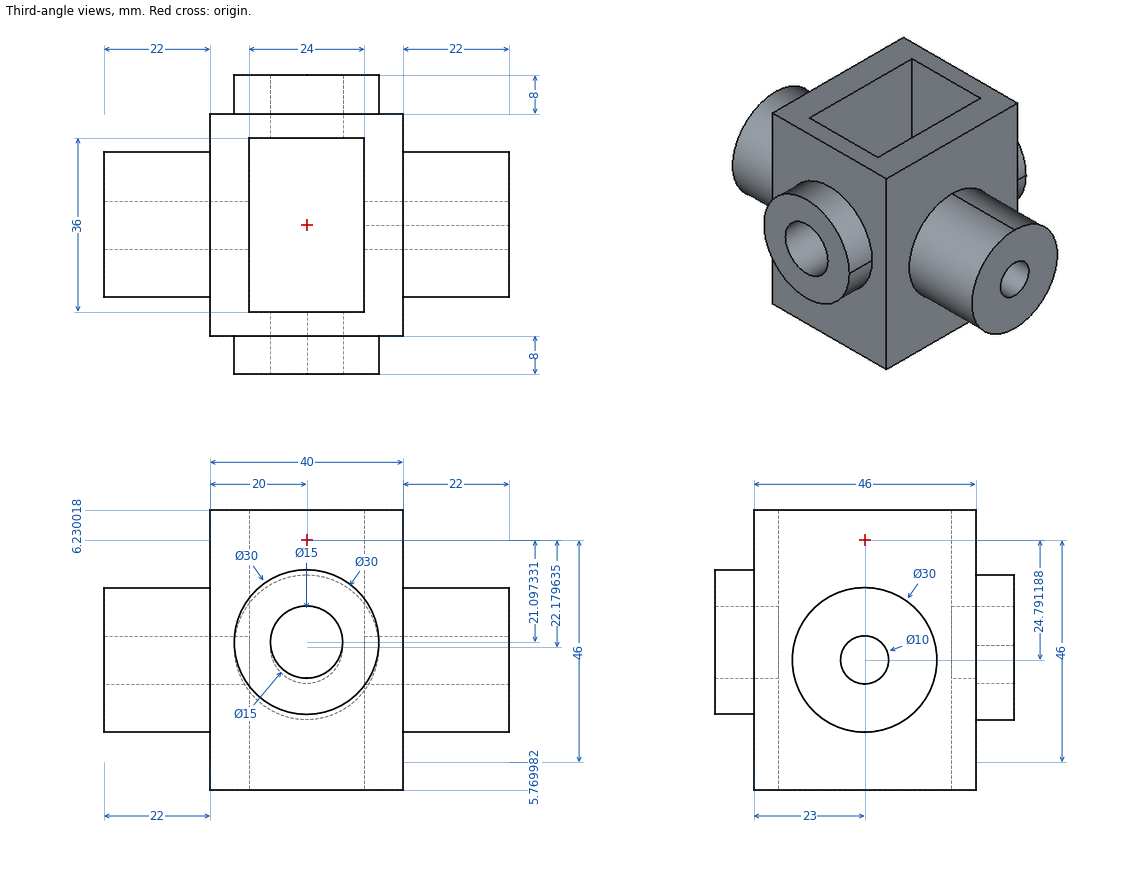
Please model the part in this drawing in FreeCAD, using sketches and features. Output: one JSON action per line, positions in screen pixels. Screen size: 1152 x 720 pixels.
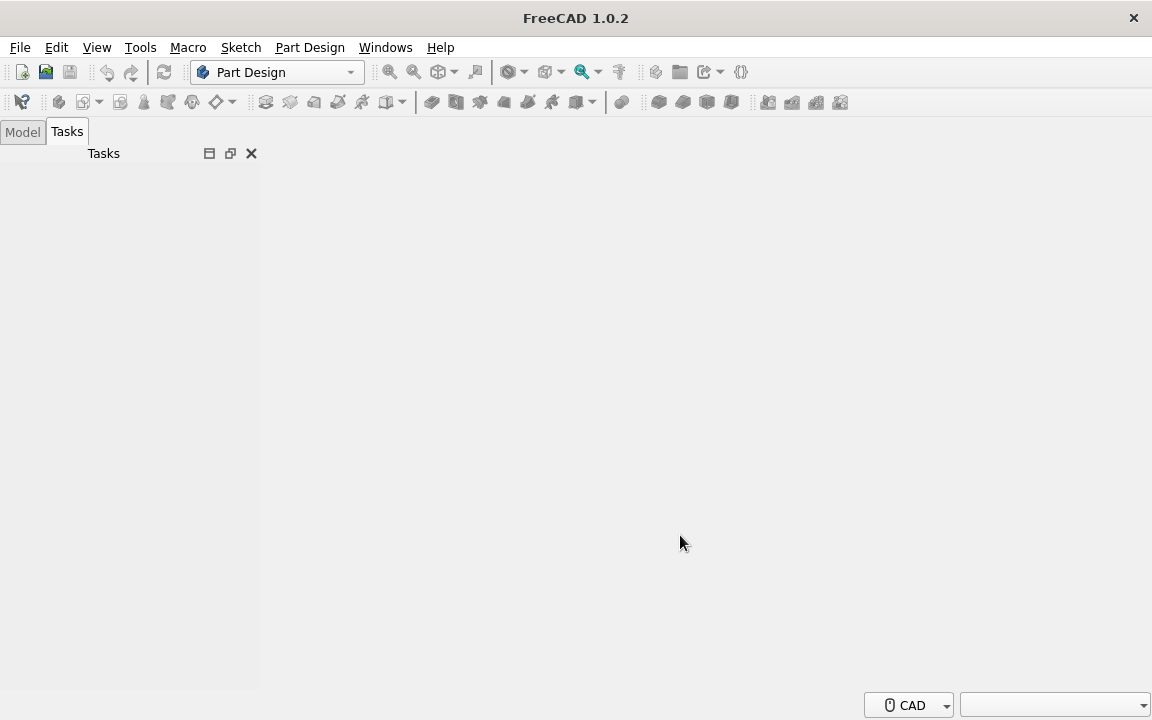
{"action": "left_click", "coordinate": [22, 72]}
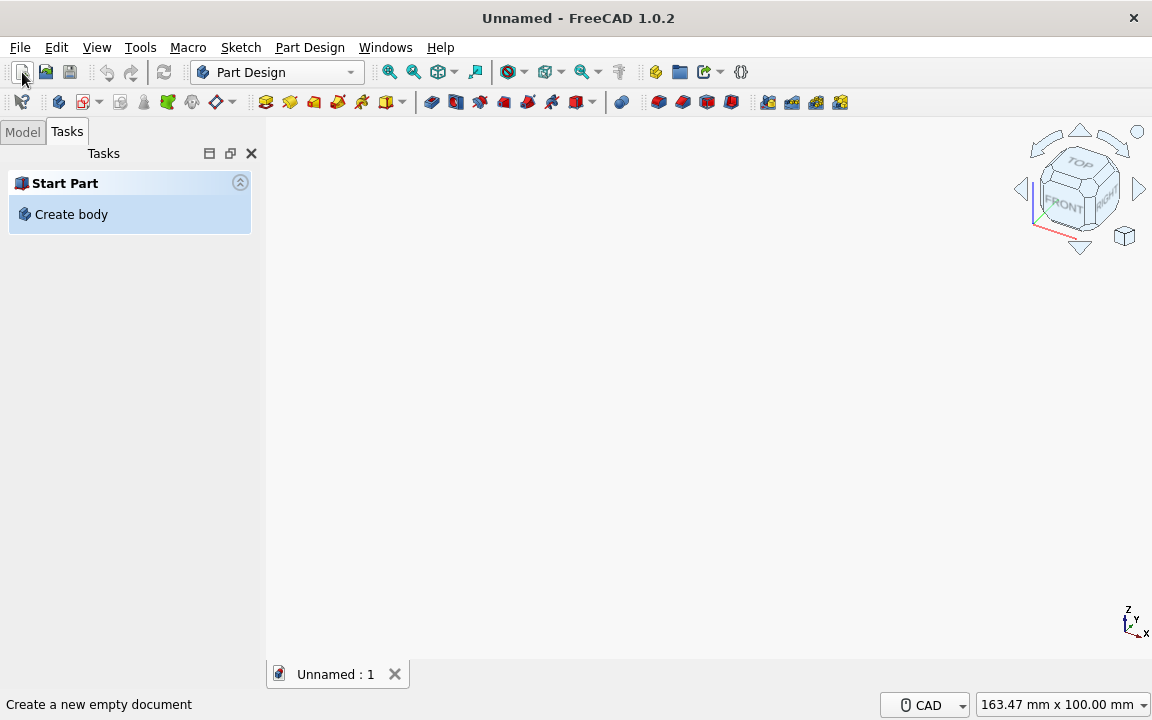
{"action": "left_click", "coordinate": [84, 102]}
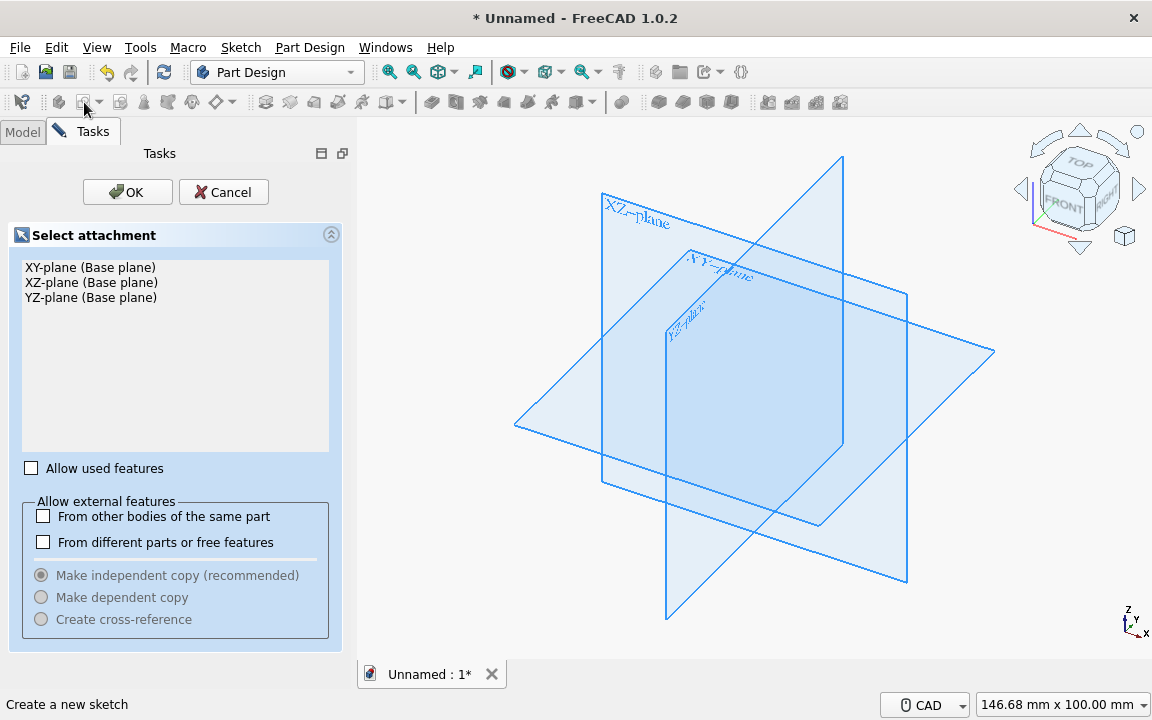
{"action": "left_click", "coordinate": [82, 282]}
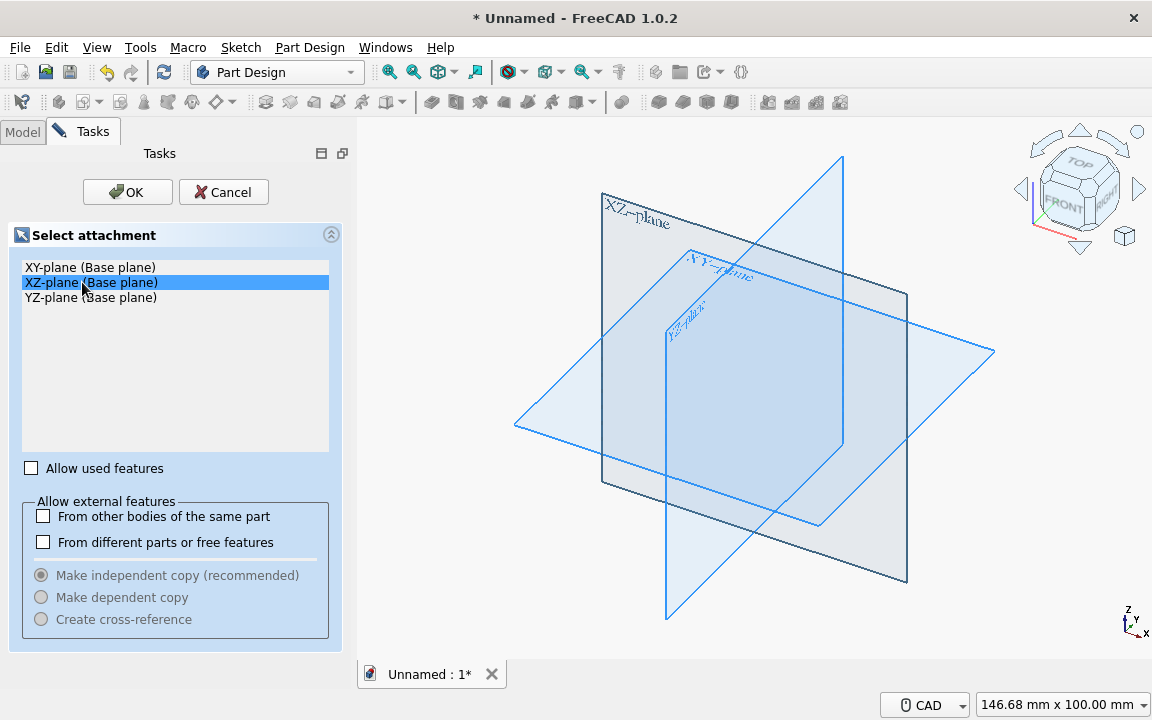
{"action": "left_click", "coordinate": [128, 192]}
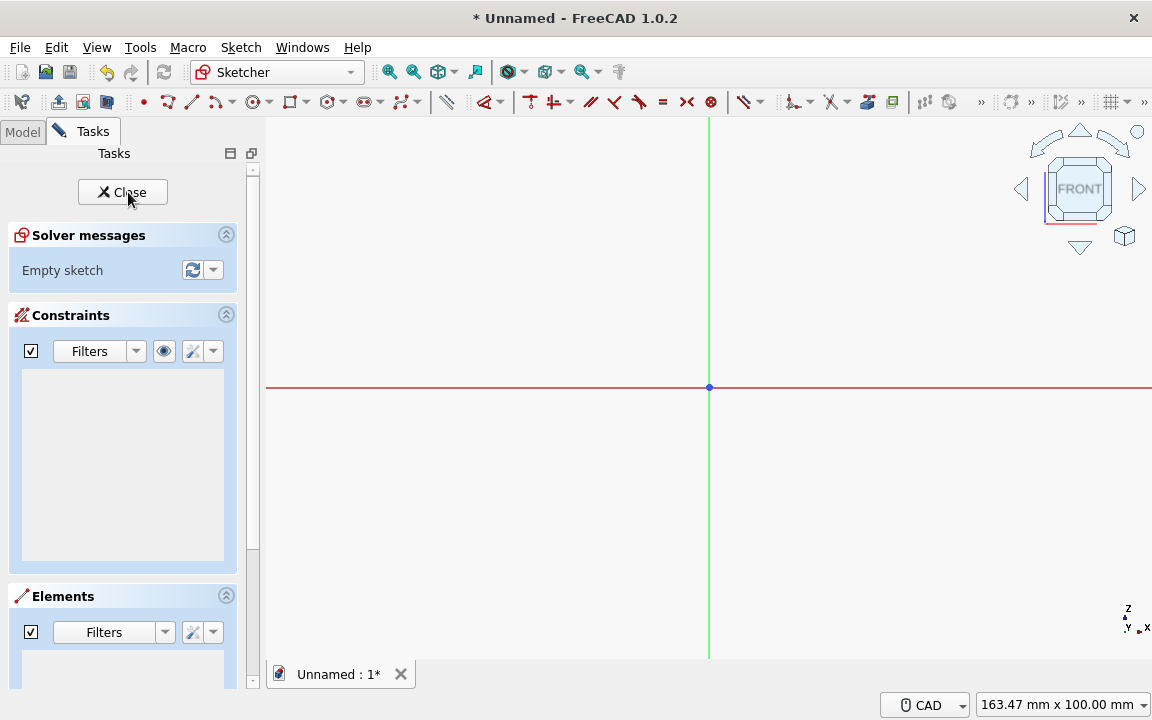
{"action": "scroll", "coordinate": [331, 145], "scroll_direction": "down", "scroll_amount": 1}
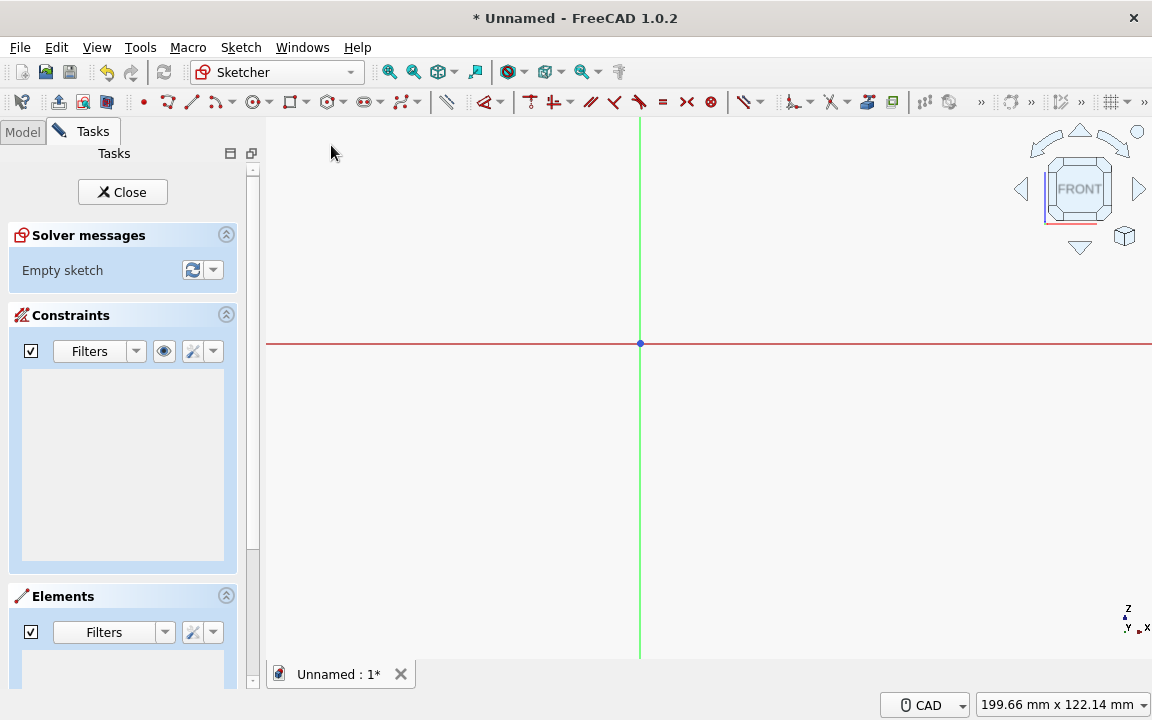
{"action": "left_click", "coordinate": [168, 102]}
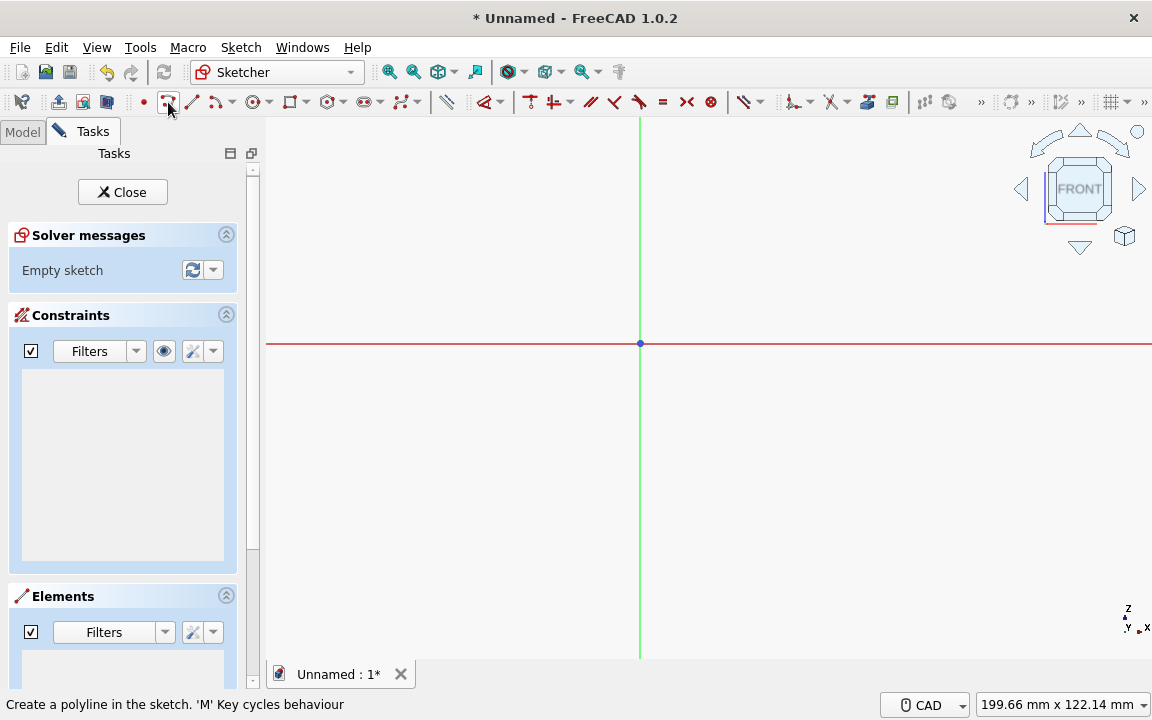
{"action": "left_click", "coordinate": [552, 344]}
{"action": "left_click", "coordinate": [552, 316]}
{"action": "left_click", "coordinate": [729, 316]}
{"action": "left_click", "coordinate": [729, 344]}
{"action": "left_click", "coordinate": [827, 353]}
{"action": "left_click", "coordinate": [827, 548]}
{"action": "left_click", "coordinate": [729, 548]}
{"action": "left_click", "coordinate": [729, 574]}
{"action": "left_click", "coordinate": [552, 574]}
{"action": "left_click", "coordinate": [552, 548]}
{"action": "left_click", "coordinate": [454, 548]}
{"action": "left_click", "coordinate": [454, 353]}
{"action": "left_click", "coordinate": [552, 344]}
{"action": "key", "text": "Escape"}
{"action": "key", "text": "Escape"}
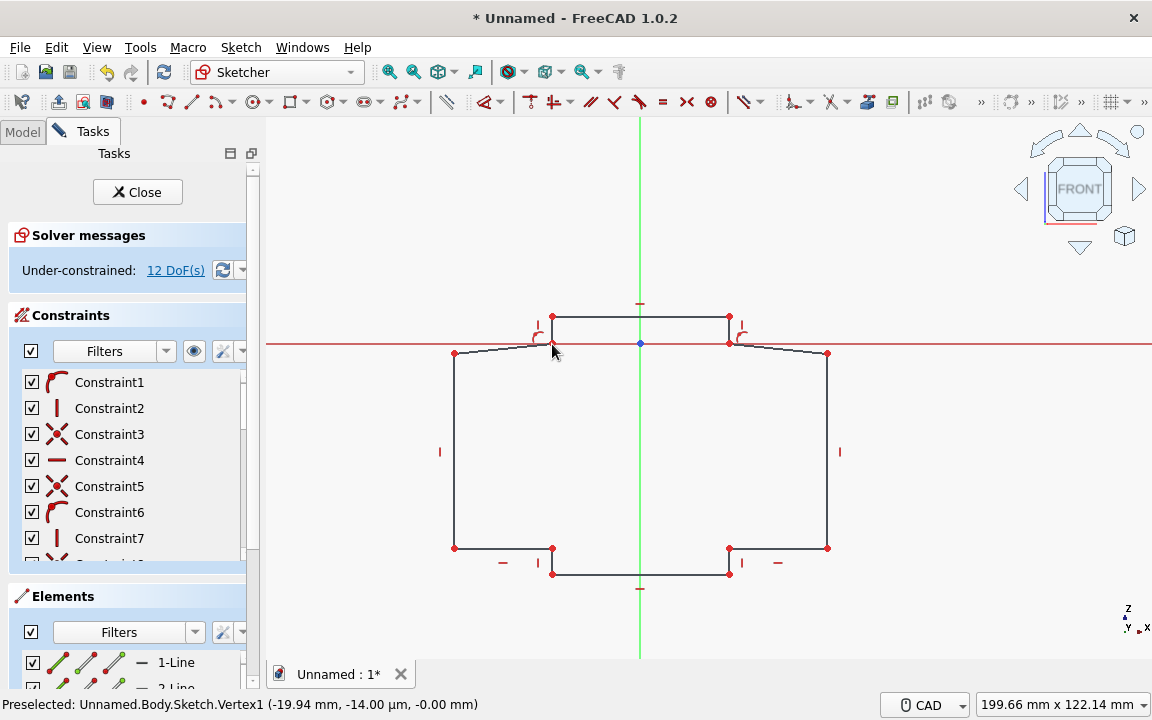
{"action": "left_click", "coordinate": [758, 347]}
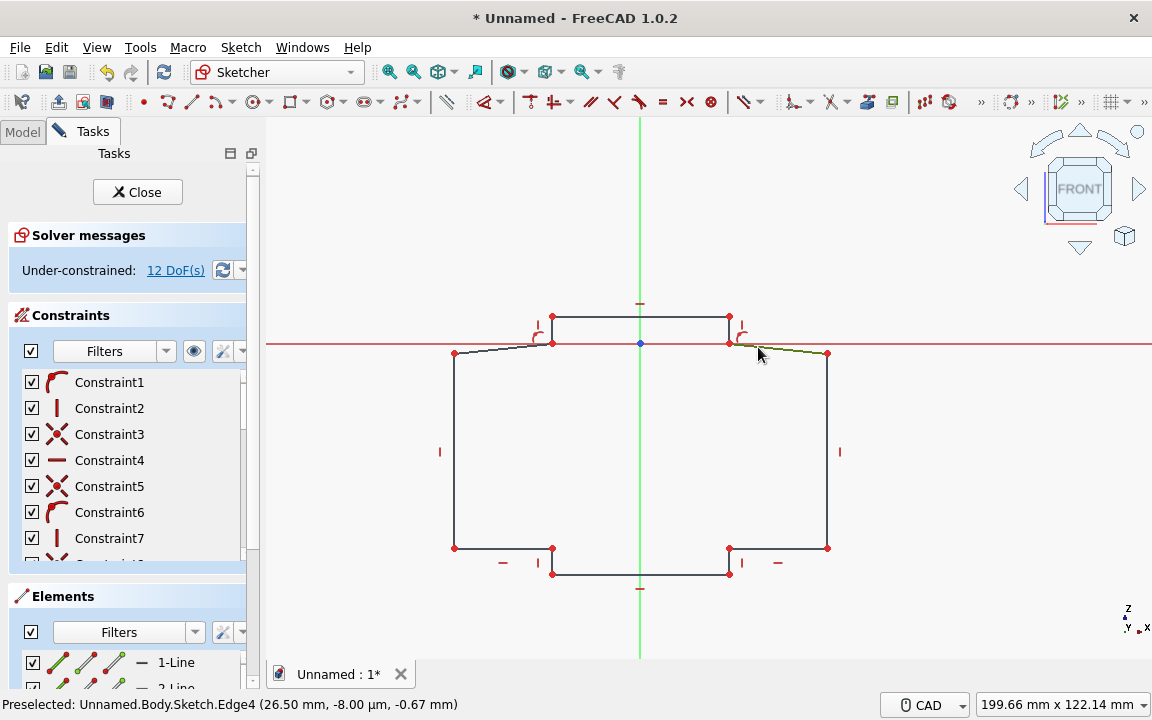
{"action": "key", "text": "h"}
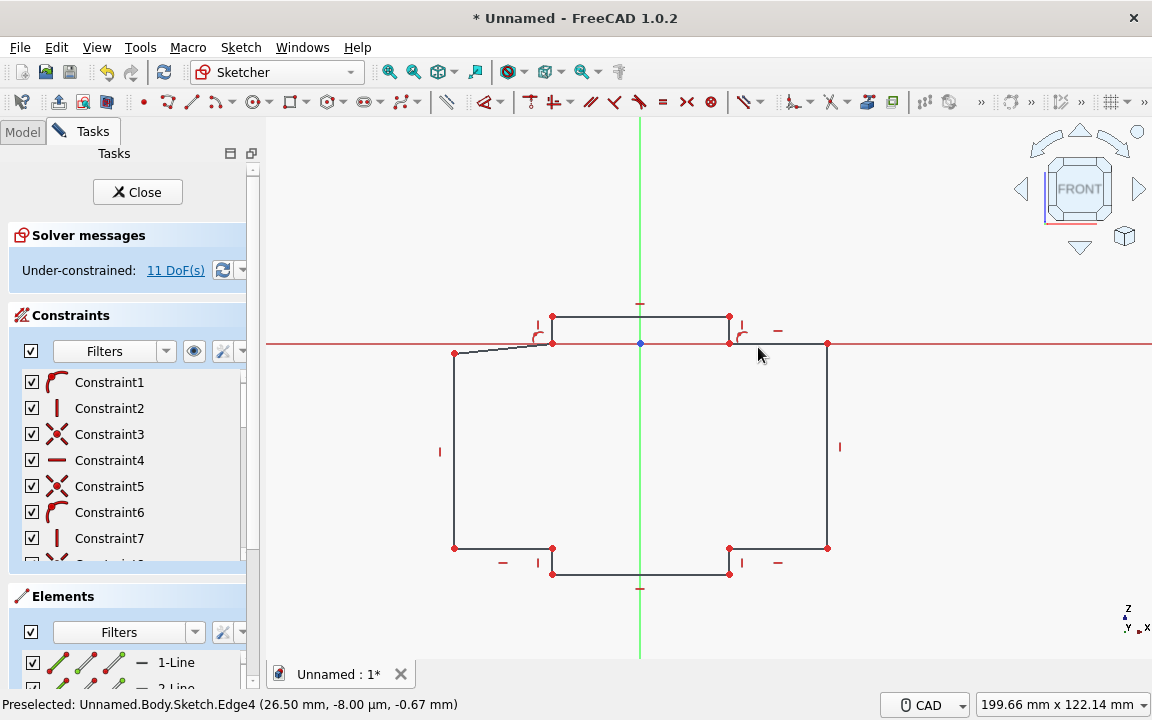
{"action": "left_click", "coordinate": [523, 347]}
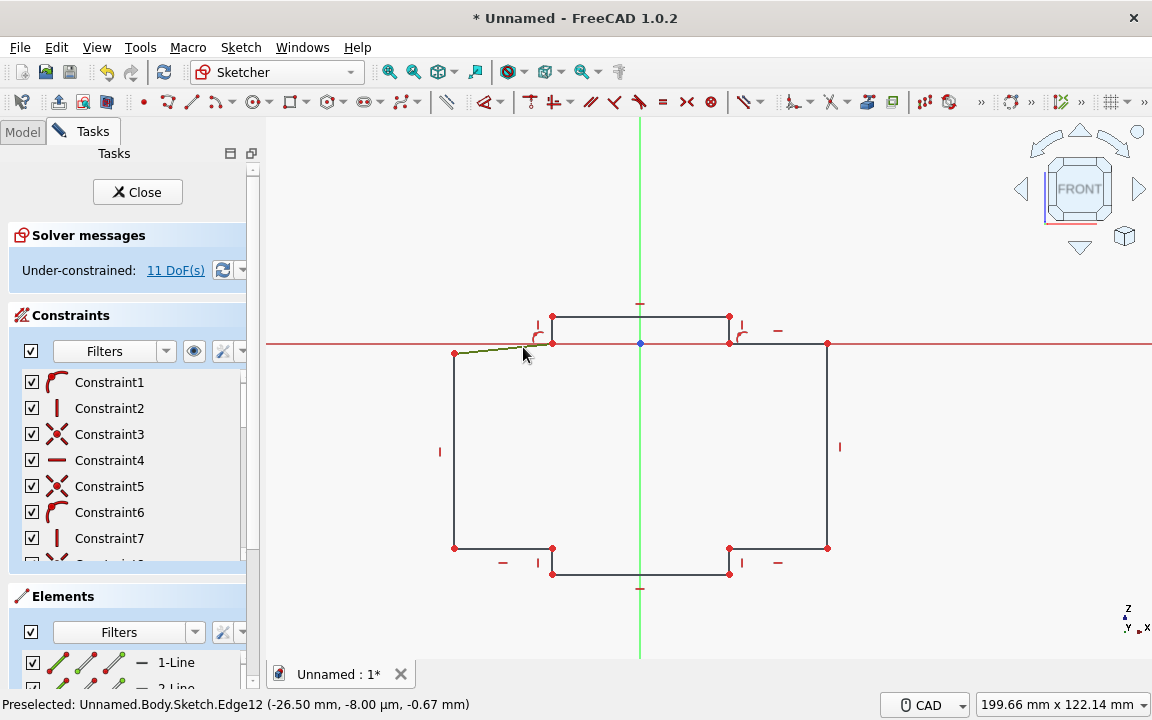
{"action": "left_click", "coordinate": [572, 102]}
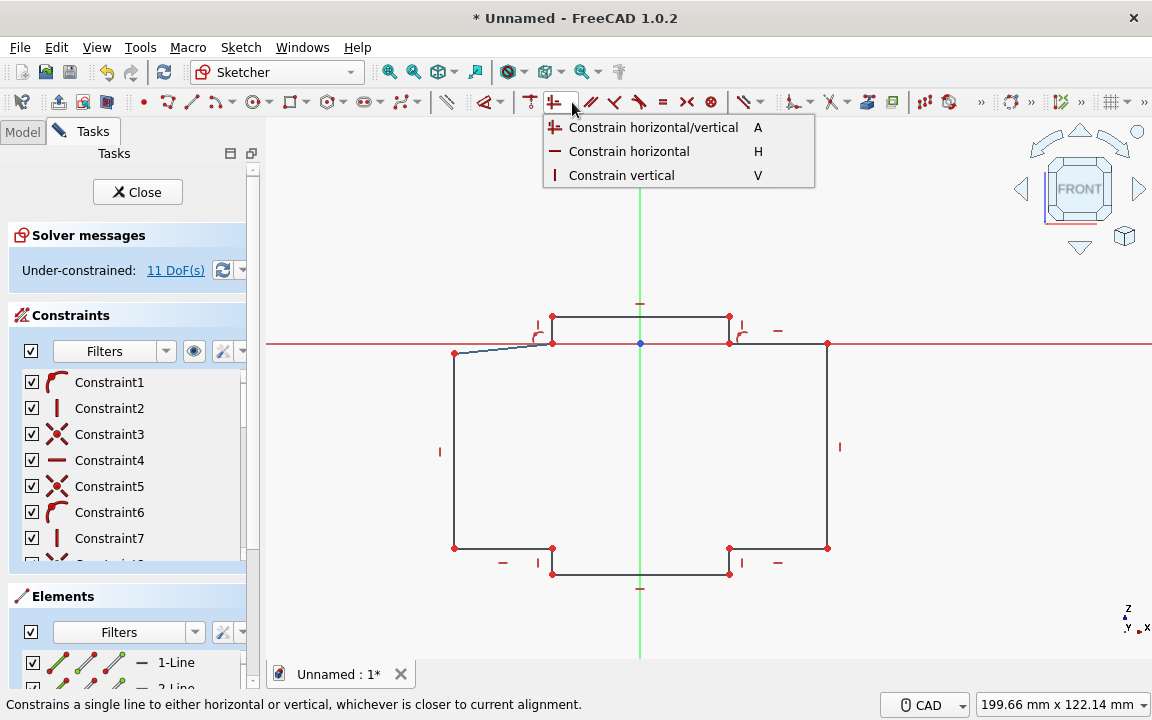
{"action": "left_click", "coordinate": [679, 151]}